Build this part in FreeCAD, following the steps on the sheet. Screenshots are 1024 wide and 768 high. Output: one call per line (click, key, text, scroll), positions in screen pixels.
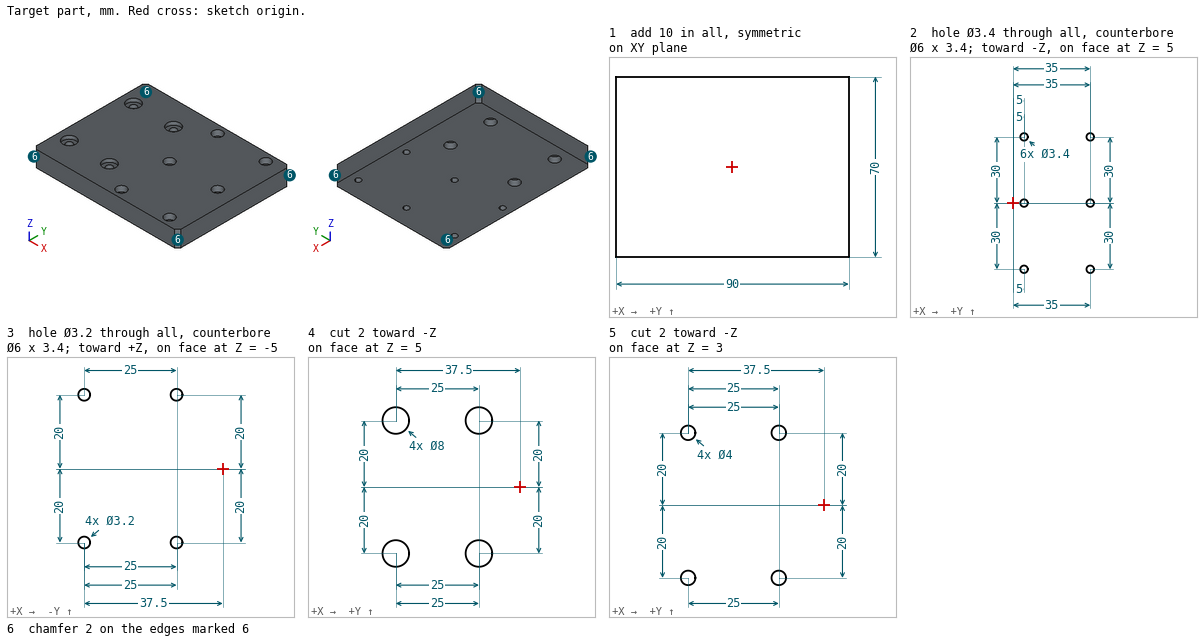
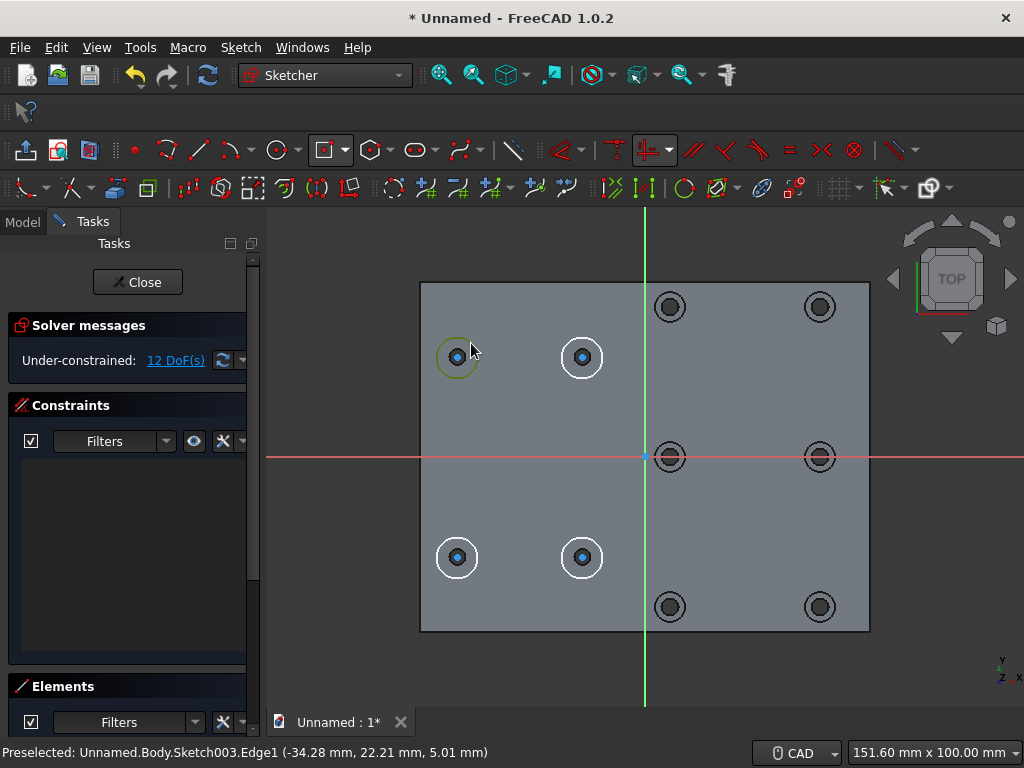
click(596, 343)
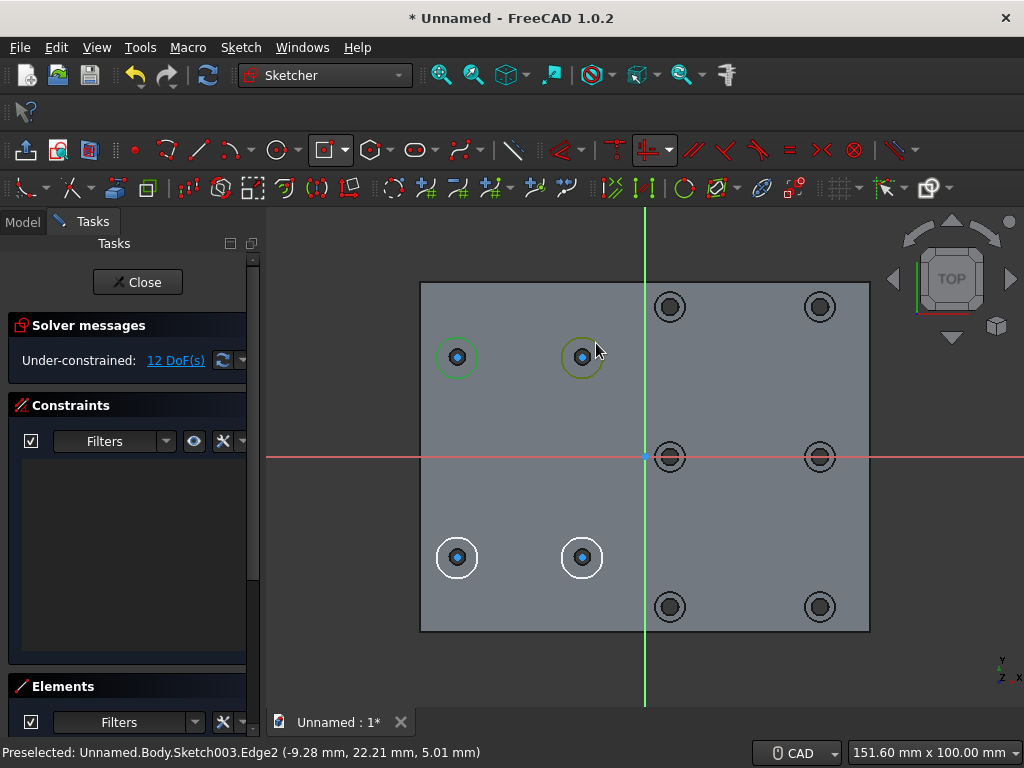
click(471, 543)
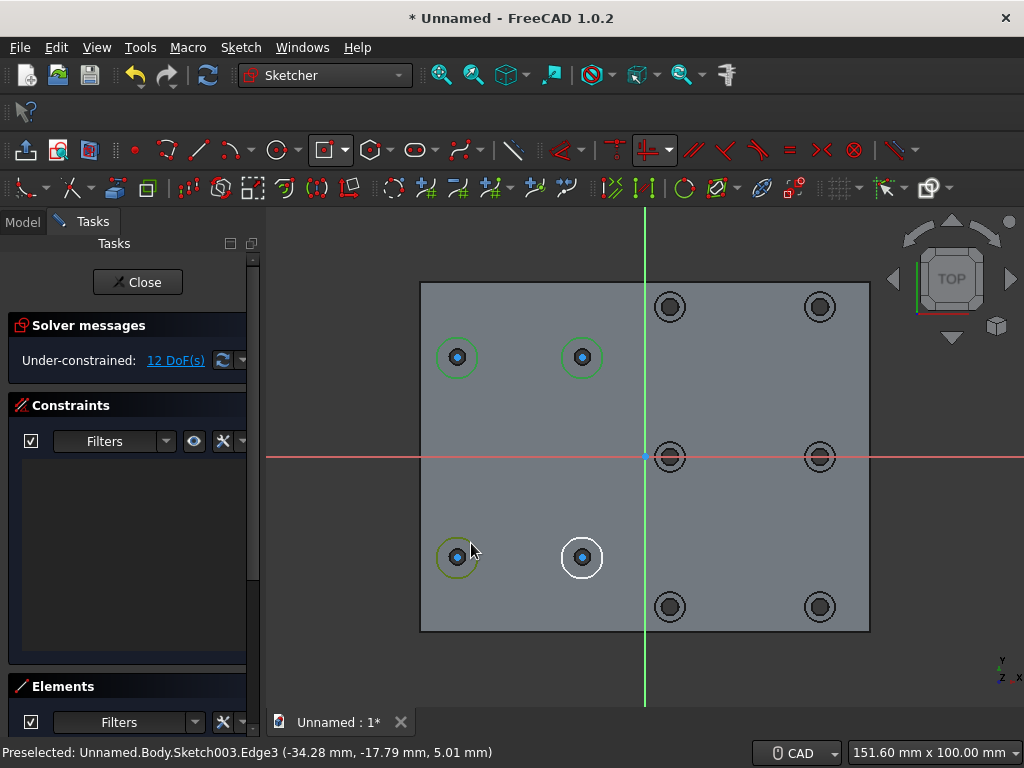
click(596, 543)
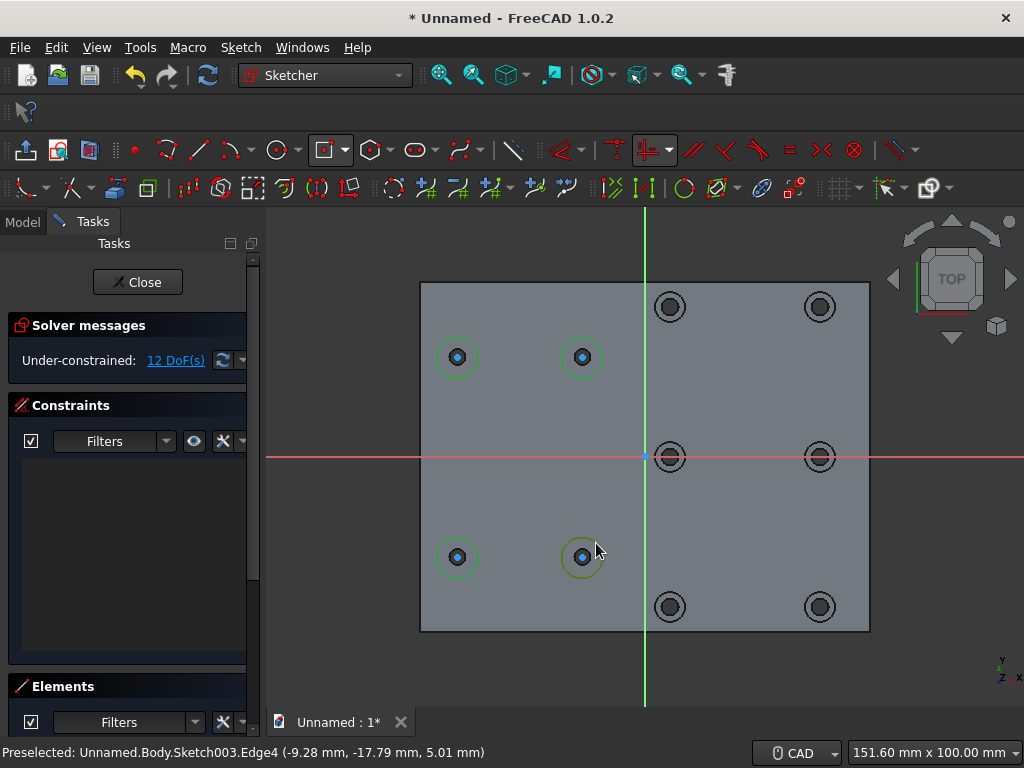
click(790, 150)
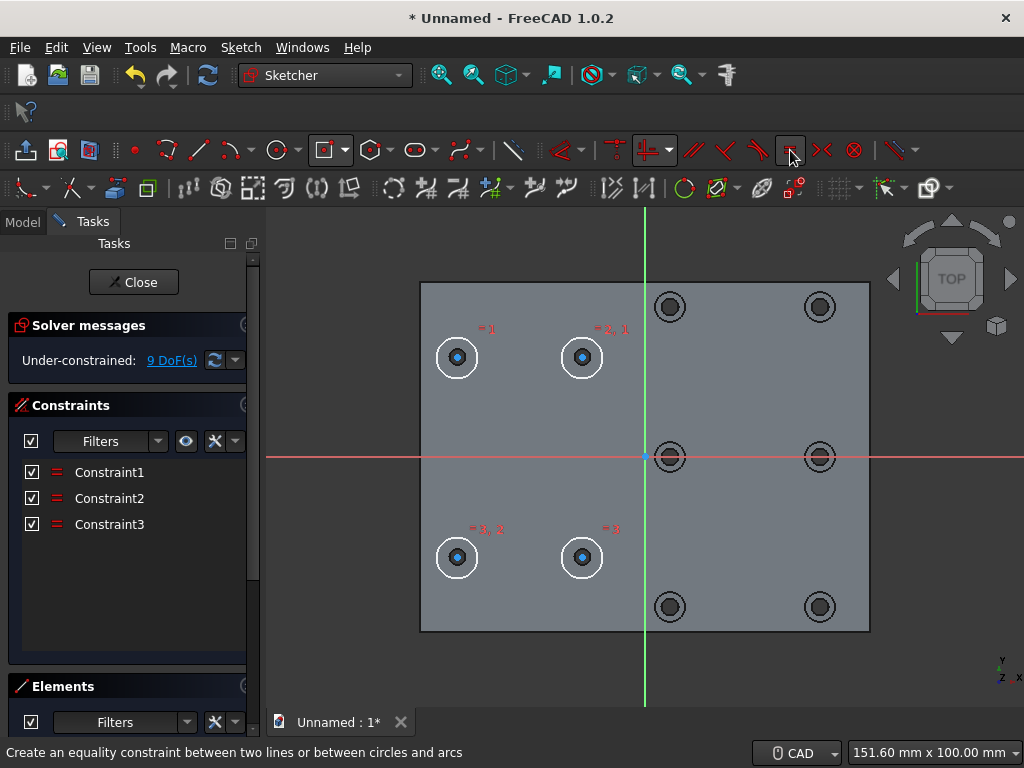
click(560, 150)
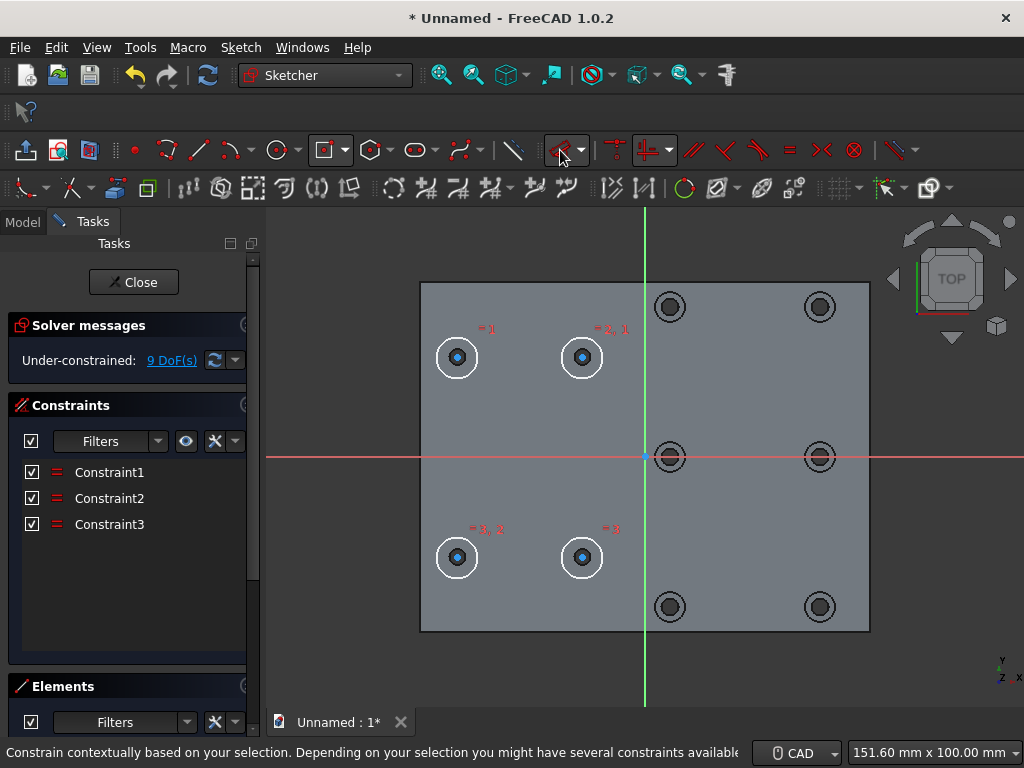
click(471, 343)
click(493, 320)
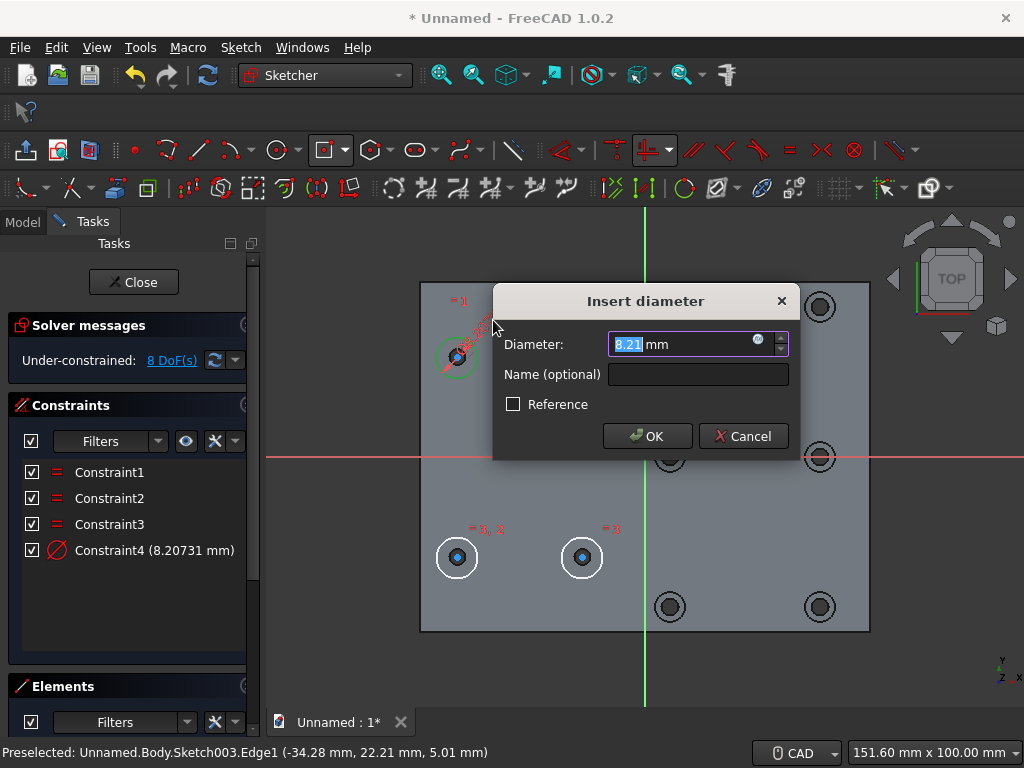
text(8)
key(Return)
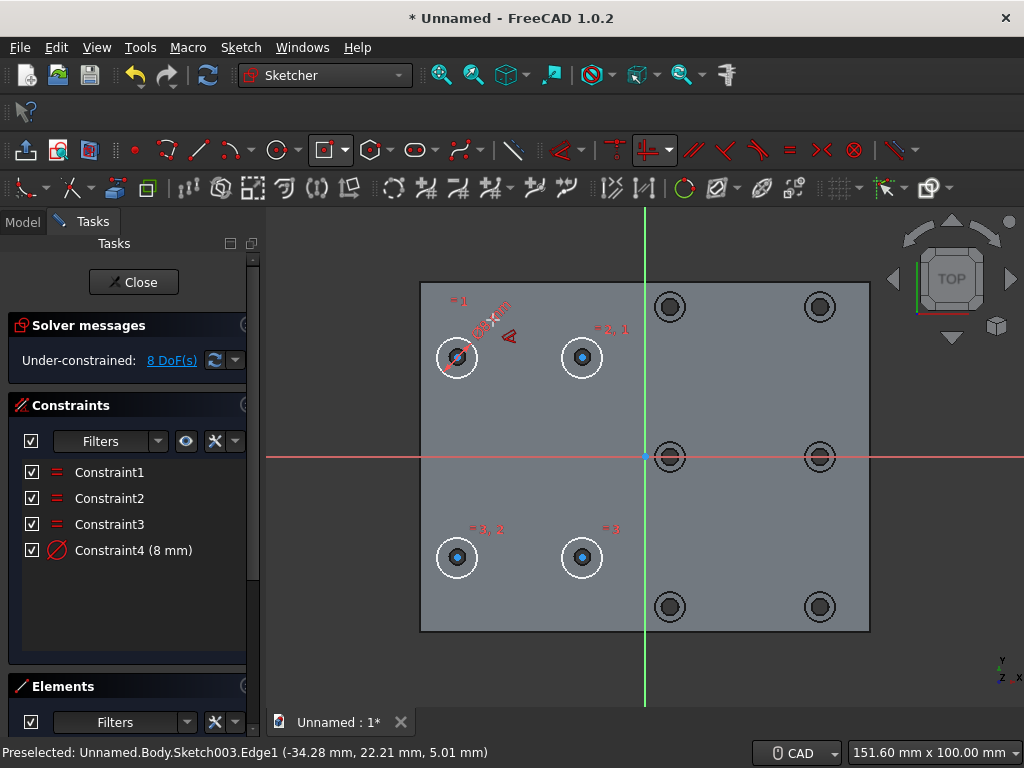
click(457, 358)
click(679, 407)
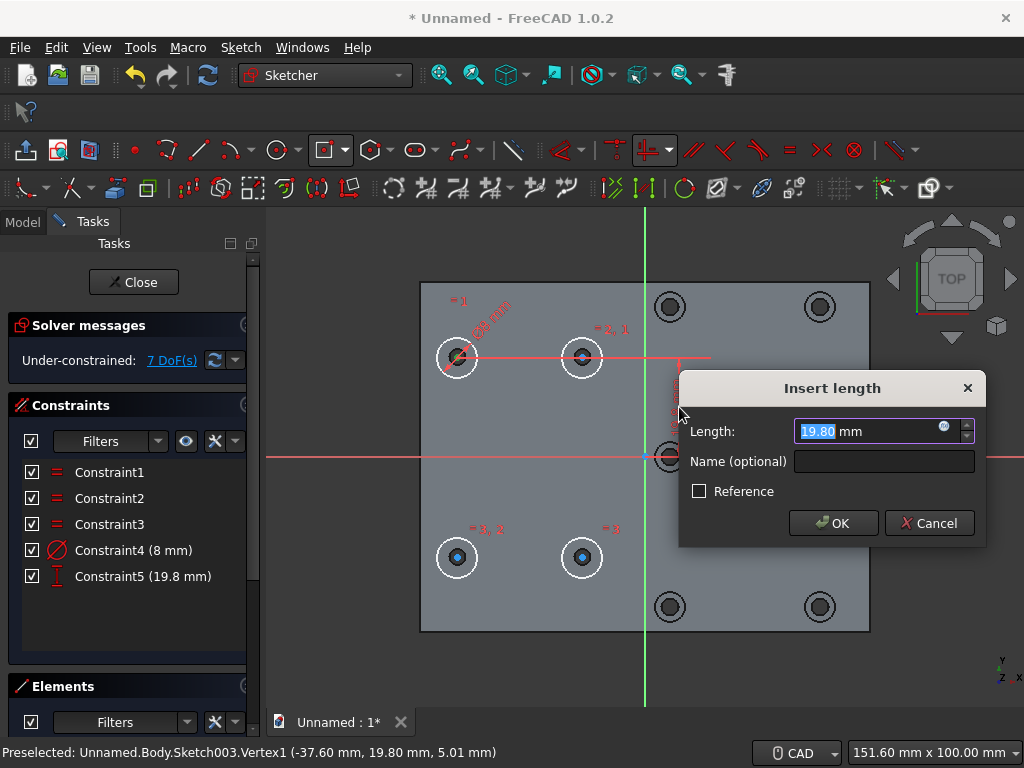
text(20)
key(Return)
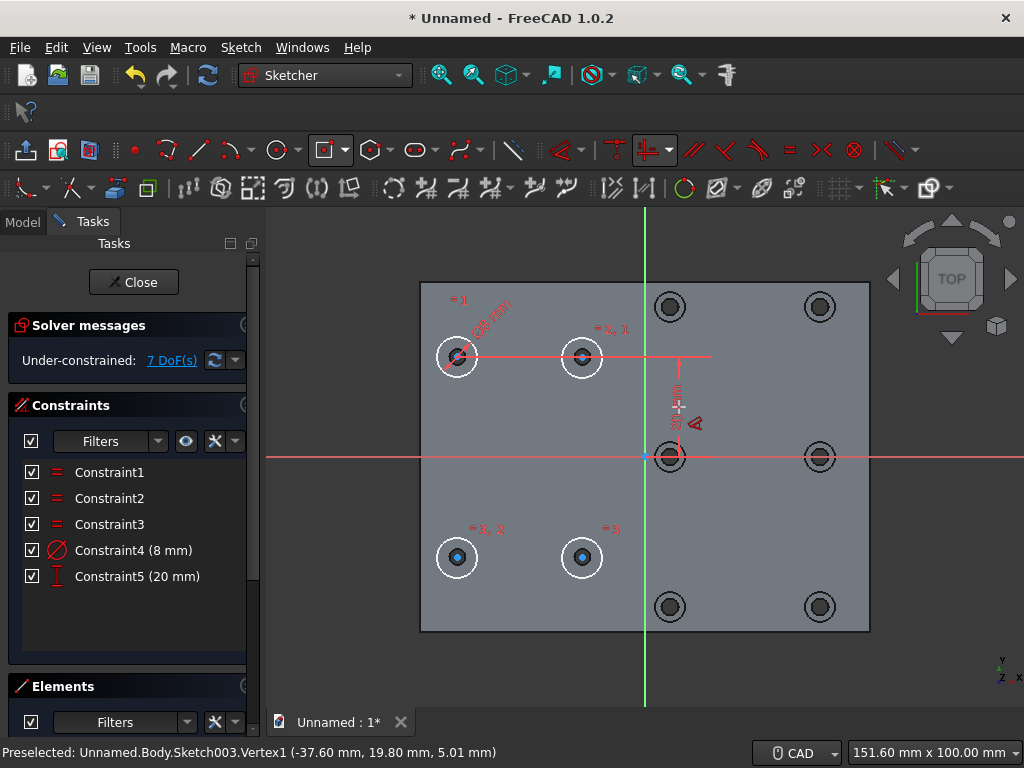
click(582, 358)
click(679, 385)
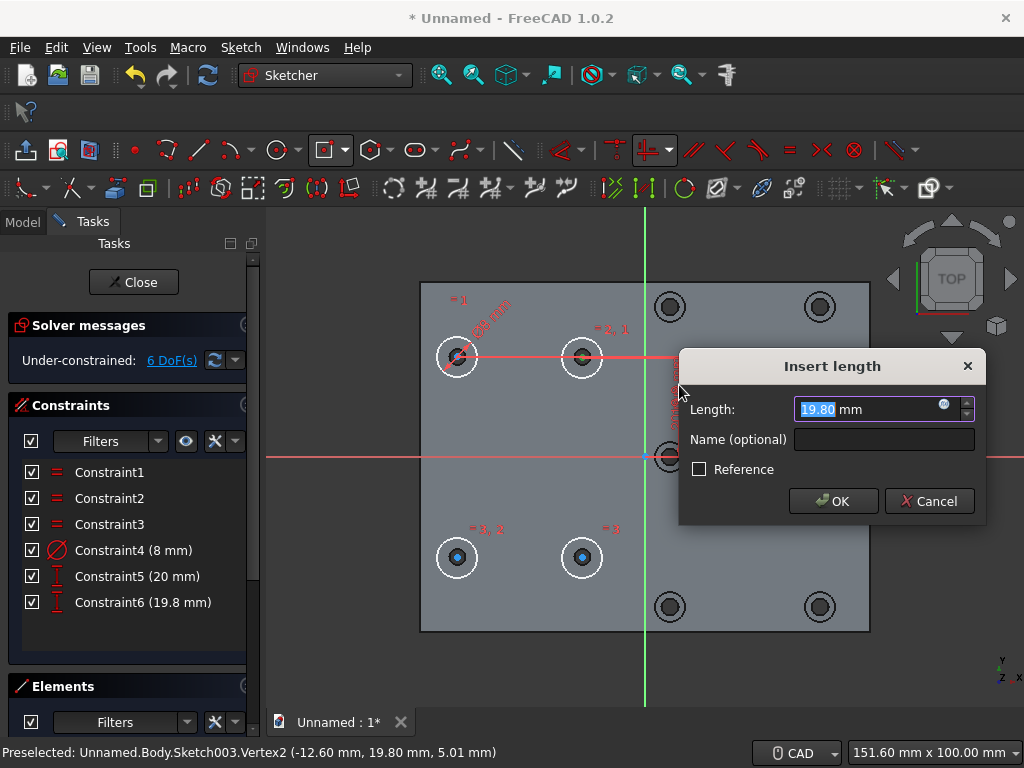
text(20)
key(Return)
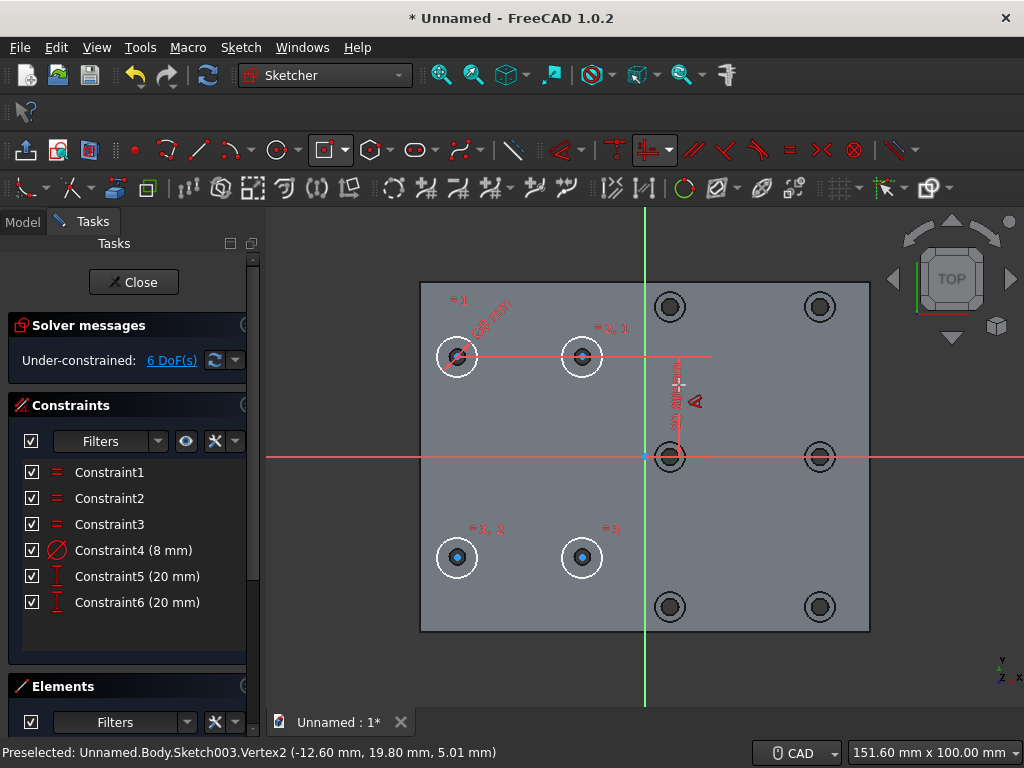
click(457, 558)
click(679, 507)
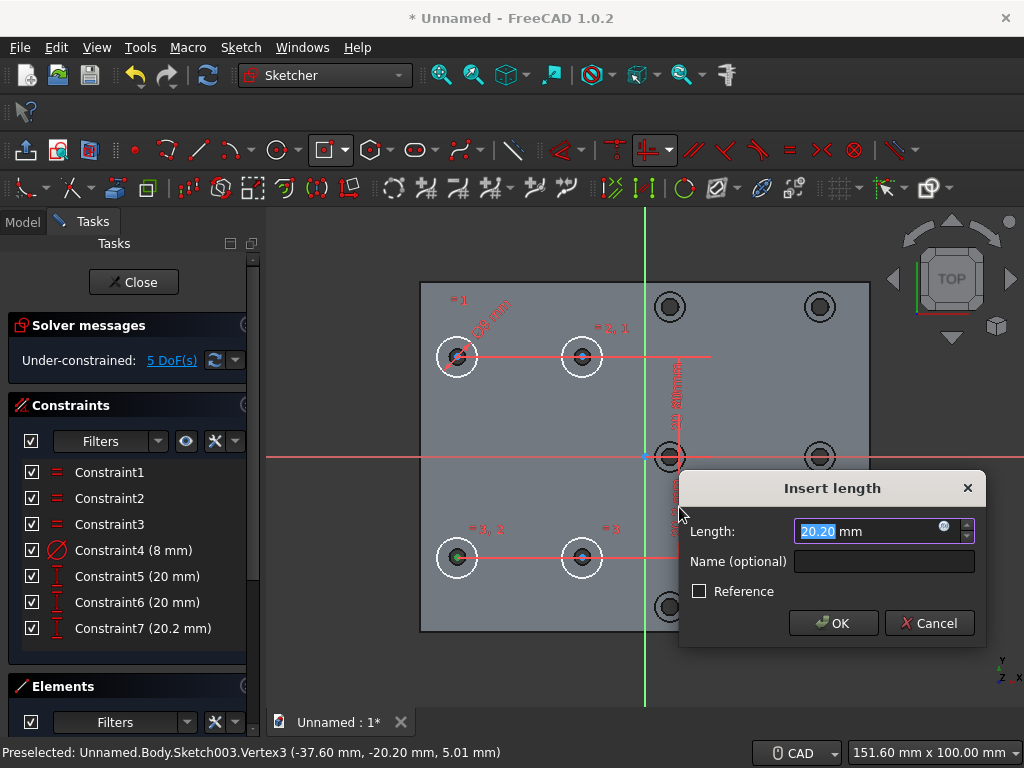
text(20)
key(Return)